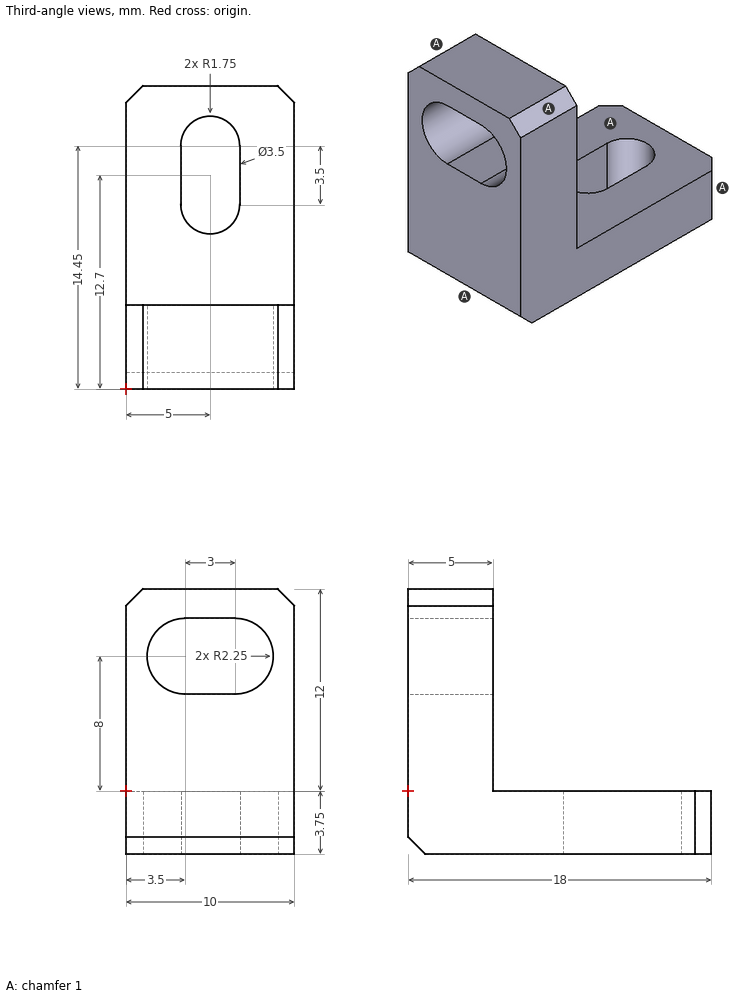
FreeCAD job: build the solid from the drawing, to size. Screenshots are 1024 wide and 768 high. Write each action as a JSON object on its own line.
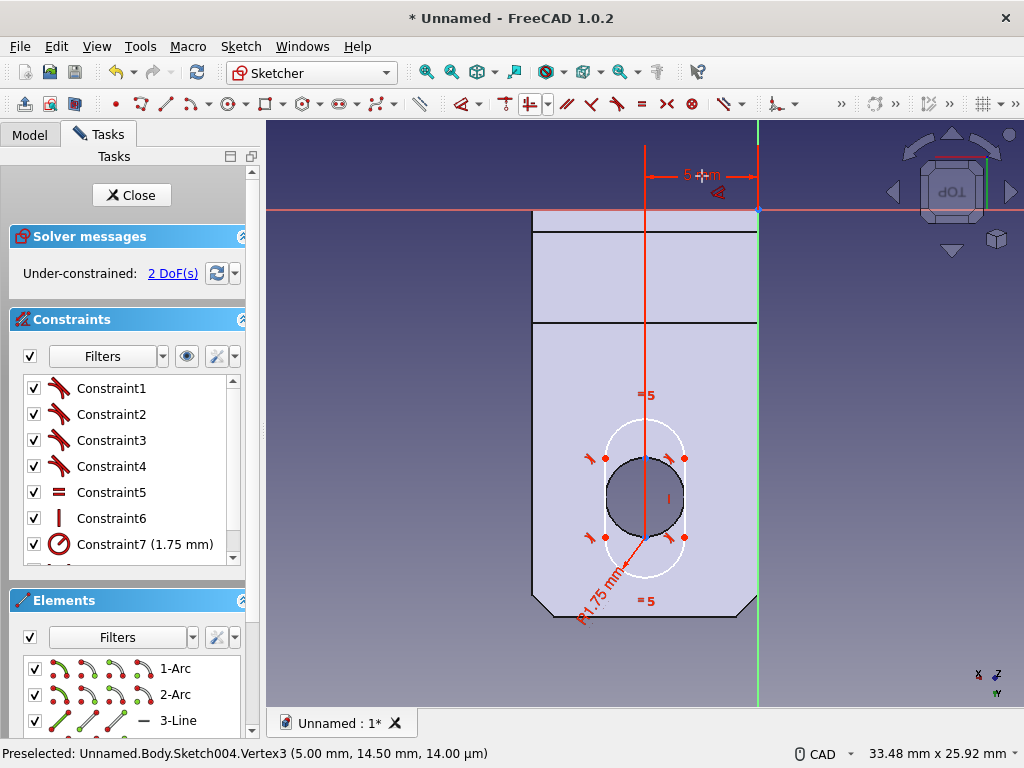
{"action": "left_click", "coordinate": [605, 514]}
{"action": "left_click", "coordinate": [571, 499]}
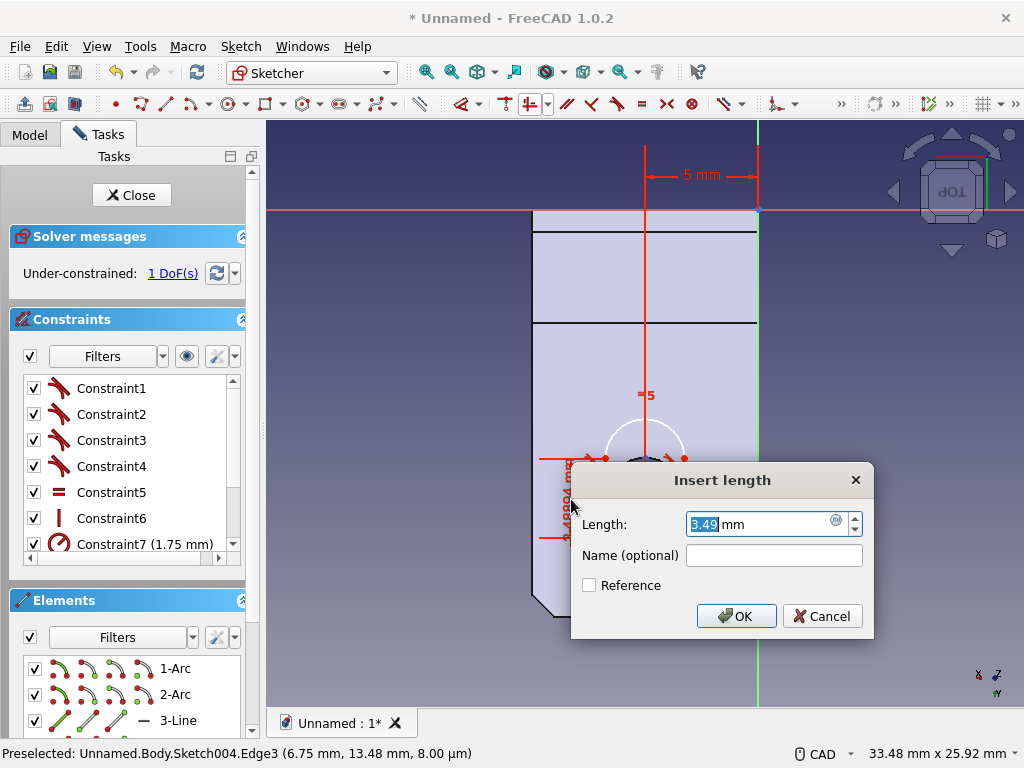
{"action": "type", "text": "3.5"}
{"action": "key", "text": "Return"}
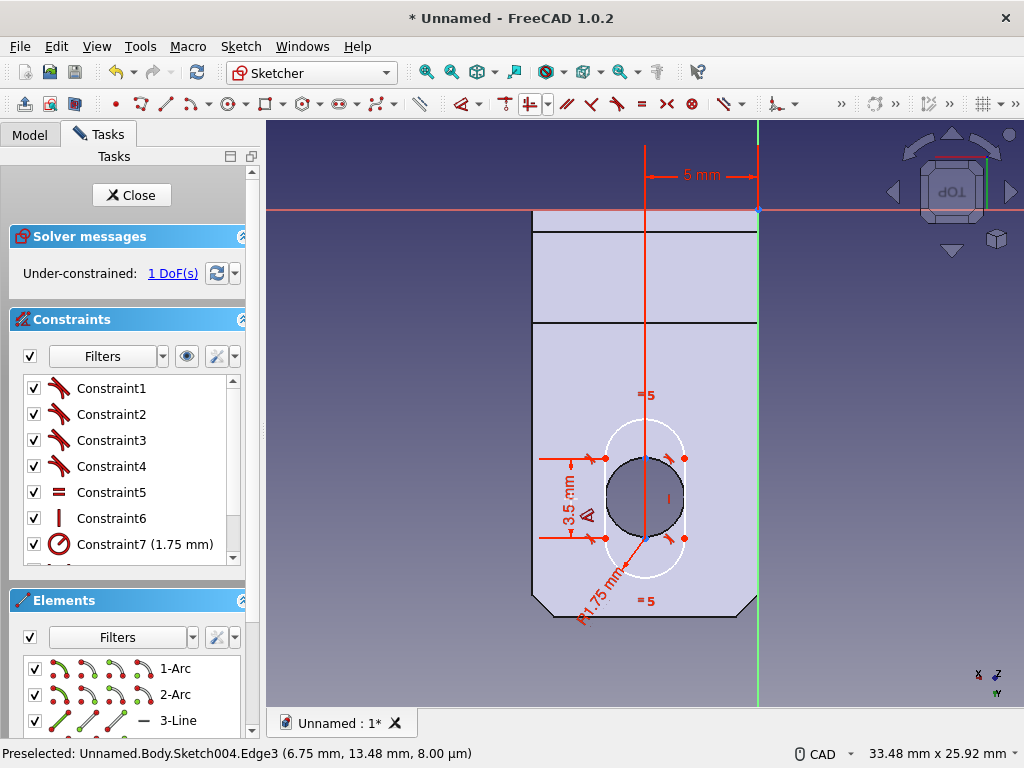
{"action": "left_click", "coordinate": [605, 538]}
{"action": "left_click", "coordinate": [792, 374]}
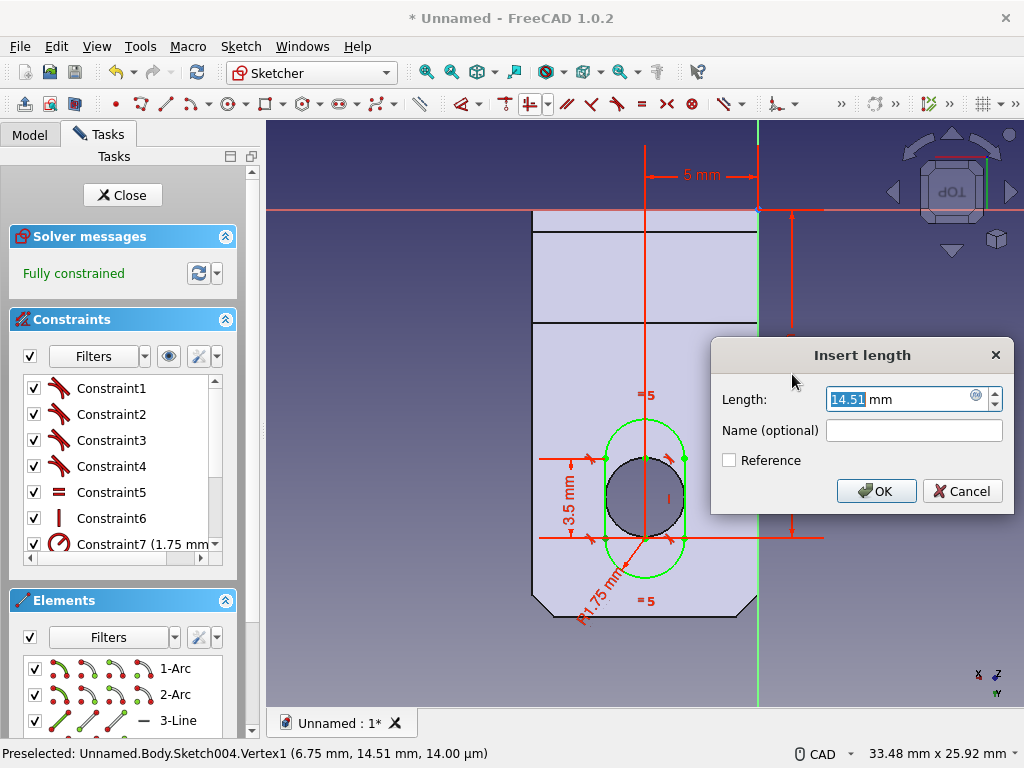
{"action": "type", "text": "14.45"}
{"action": "key", "text": "Return"}
{"action": "key", "text": "Escape"}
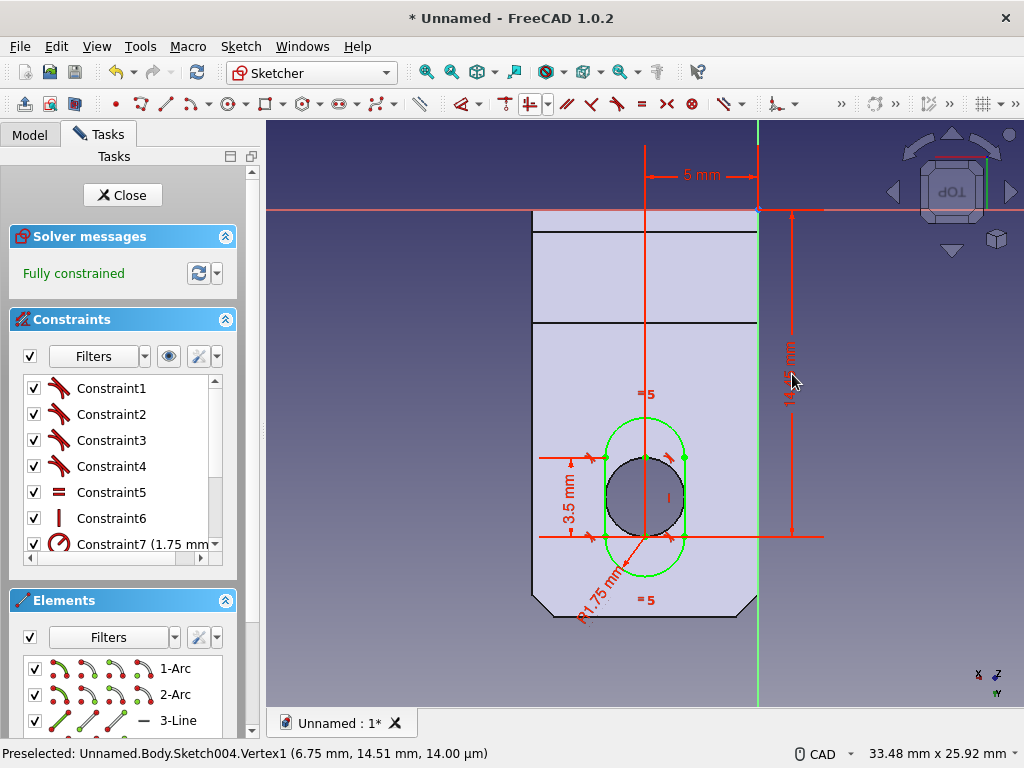
{"action": "left_click", "coordinate": [123, 195]}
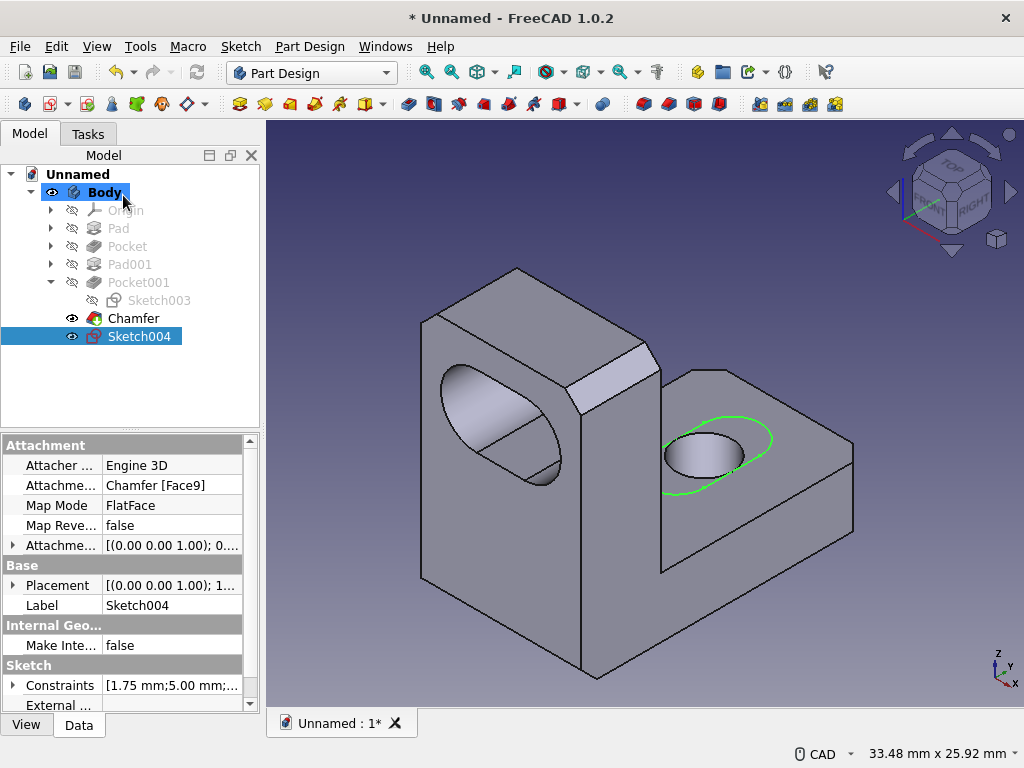
{"action": "left_click", "coordinate": [409, 104]}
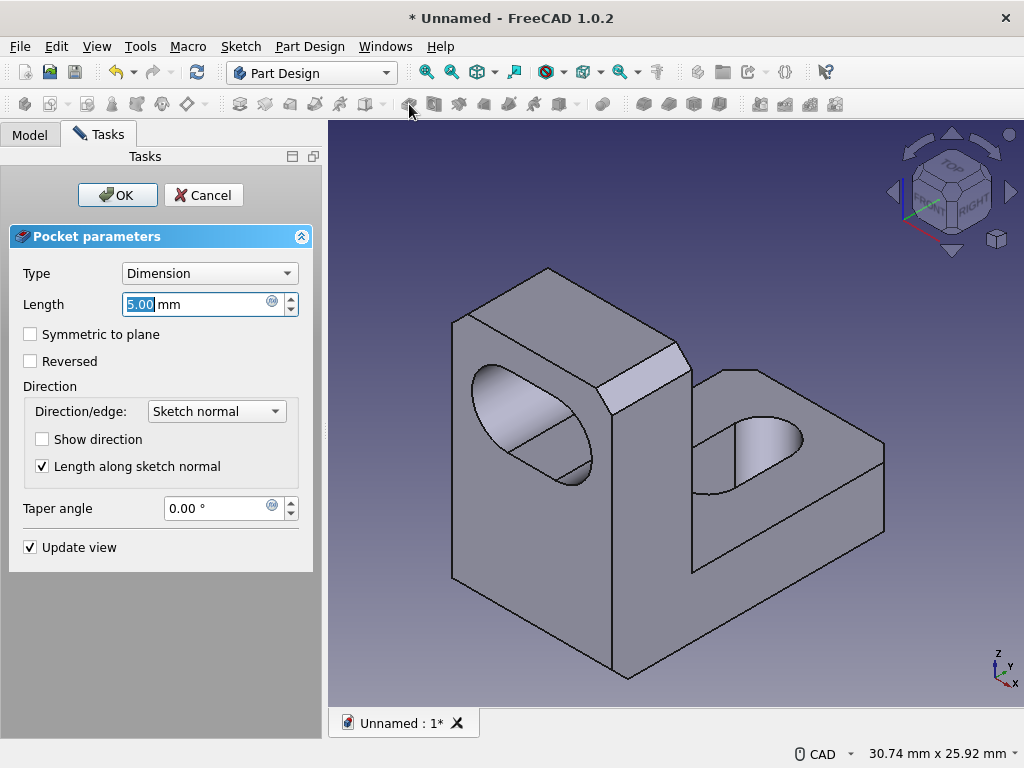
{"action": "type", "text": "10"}
{"action": "key", "text": "Tab"}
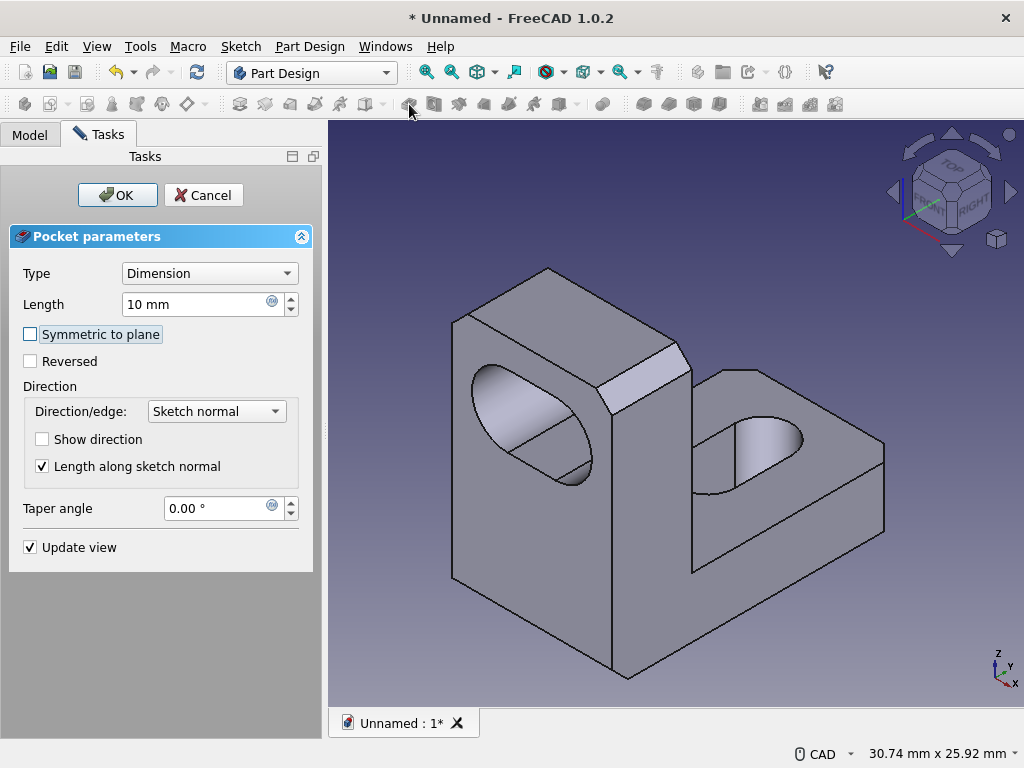
{"action": "left_click", "coordinate": [118, 195]}